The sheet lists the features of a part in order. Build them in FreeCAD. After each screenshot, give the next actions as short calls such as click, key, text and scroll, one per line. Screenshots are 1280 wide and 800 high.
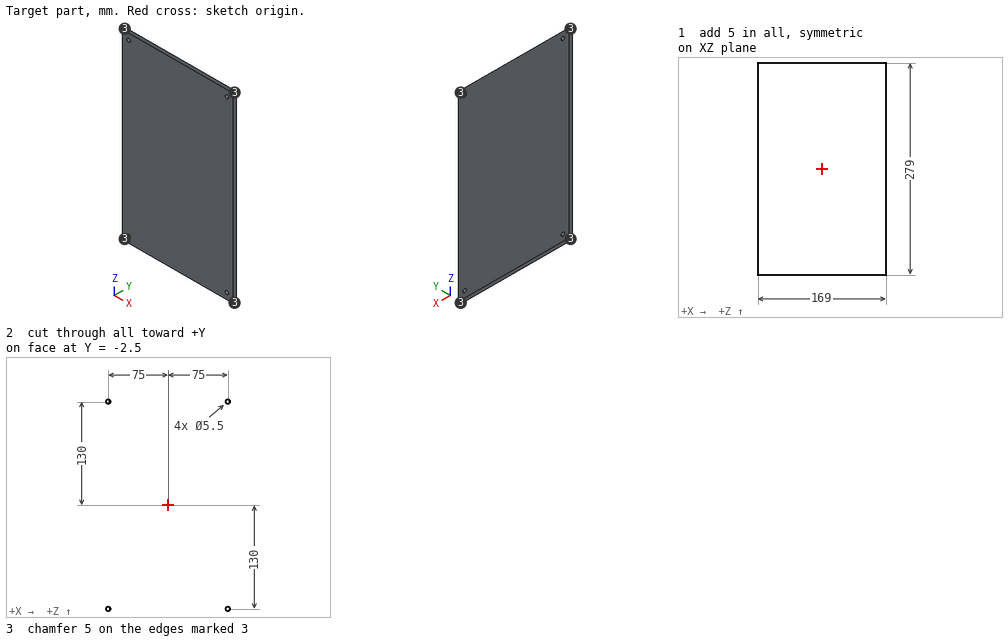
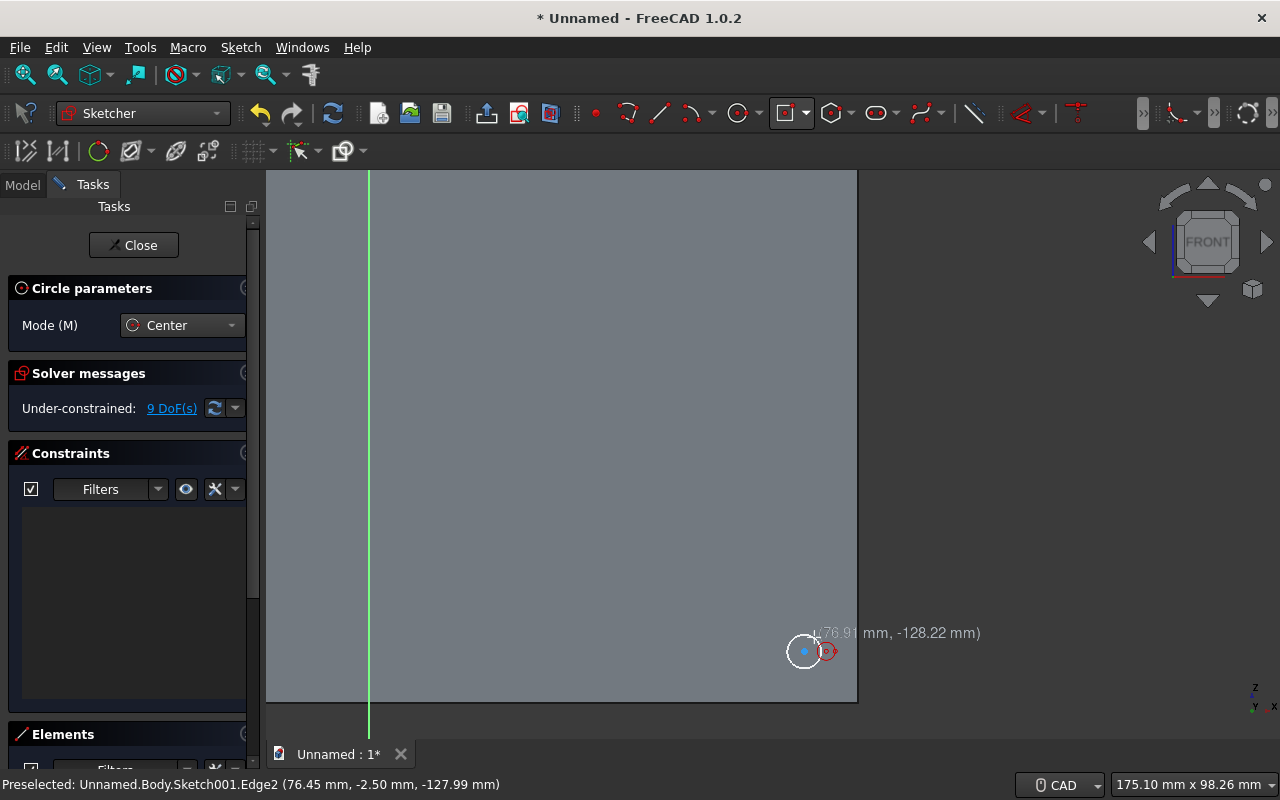
scroll(814, 637, down, 7)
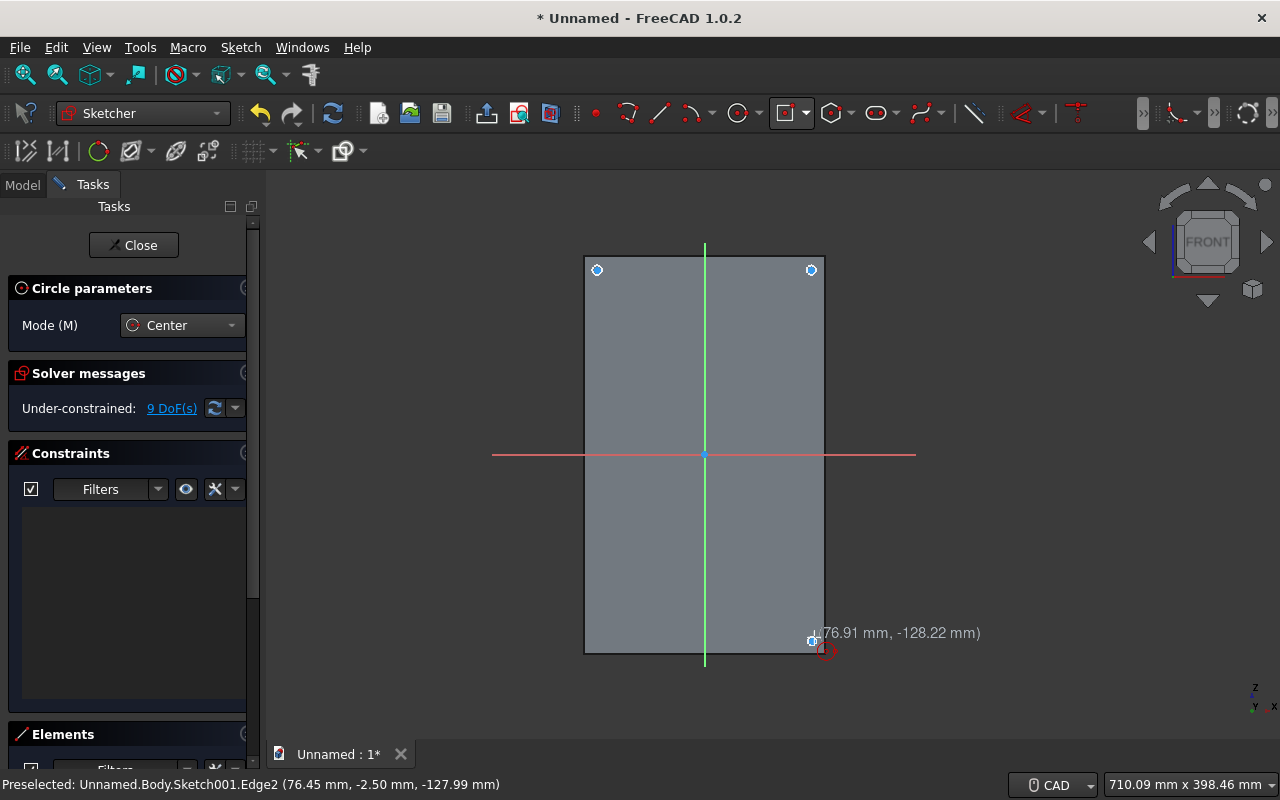
scroll(597, 640, up, 9)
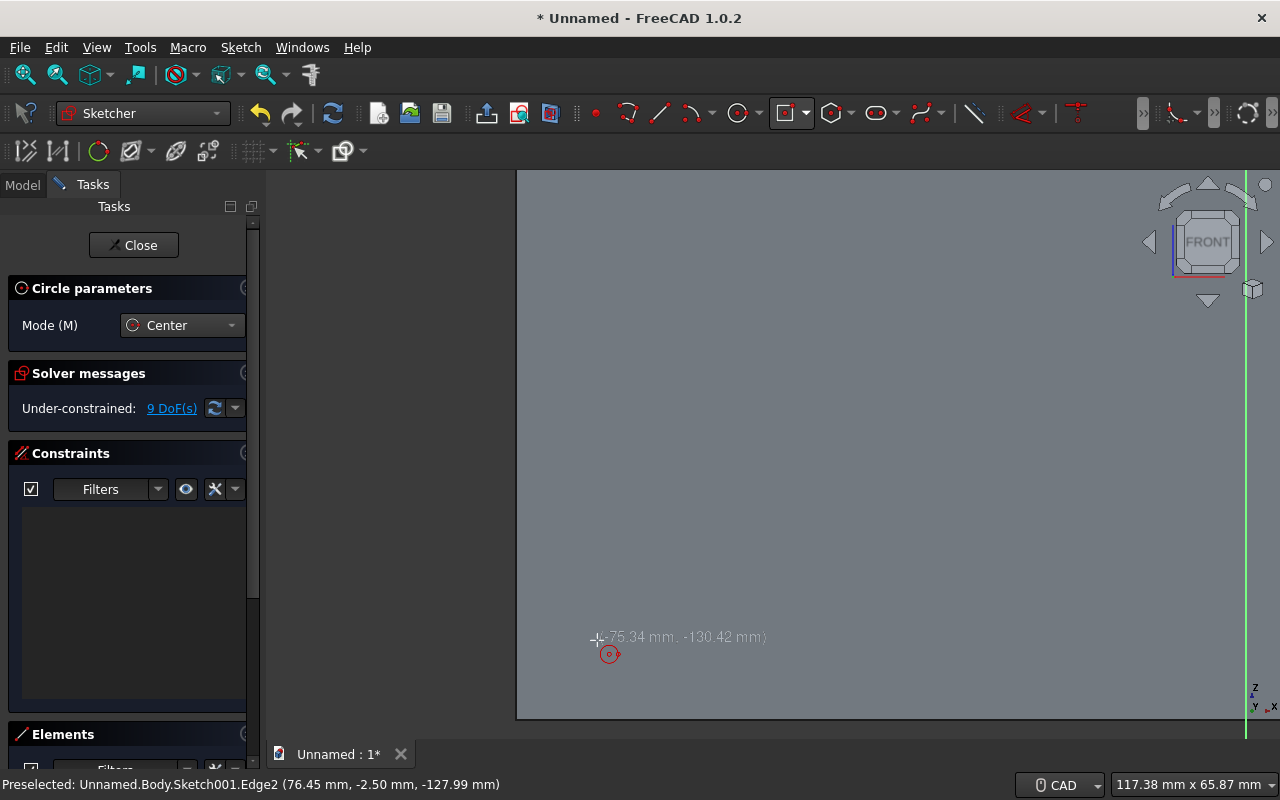
scroll(597, 641, down, 9)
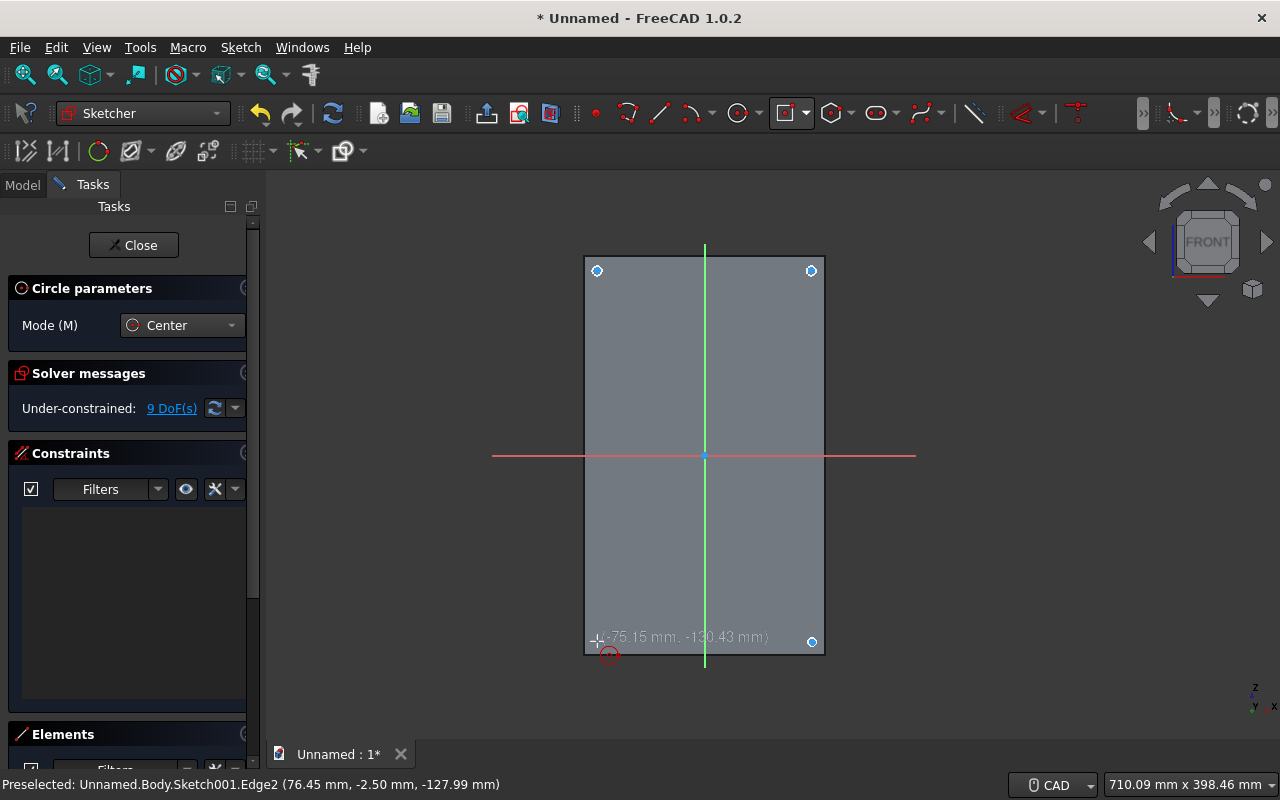
click(597, 641)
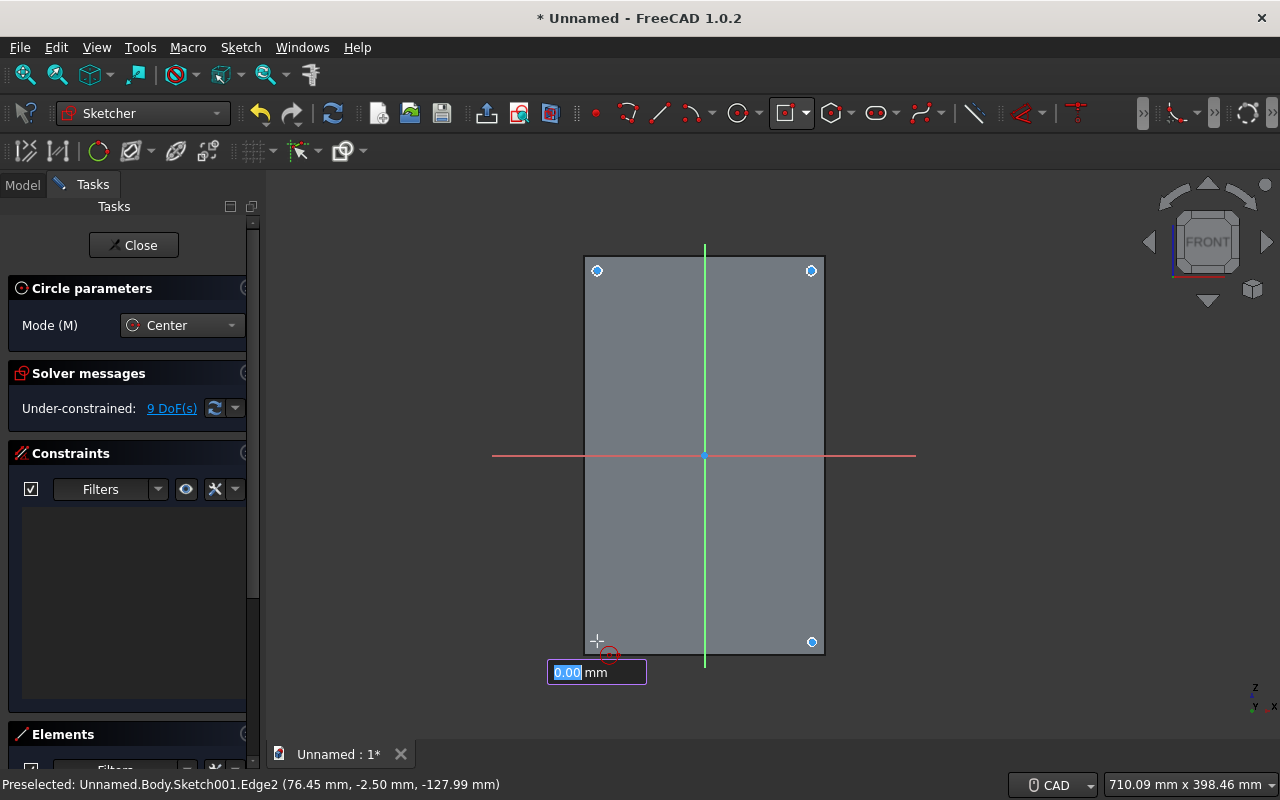
scroll(600, 638, up, 7)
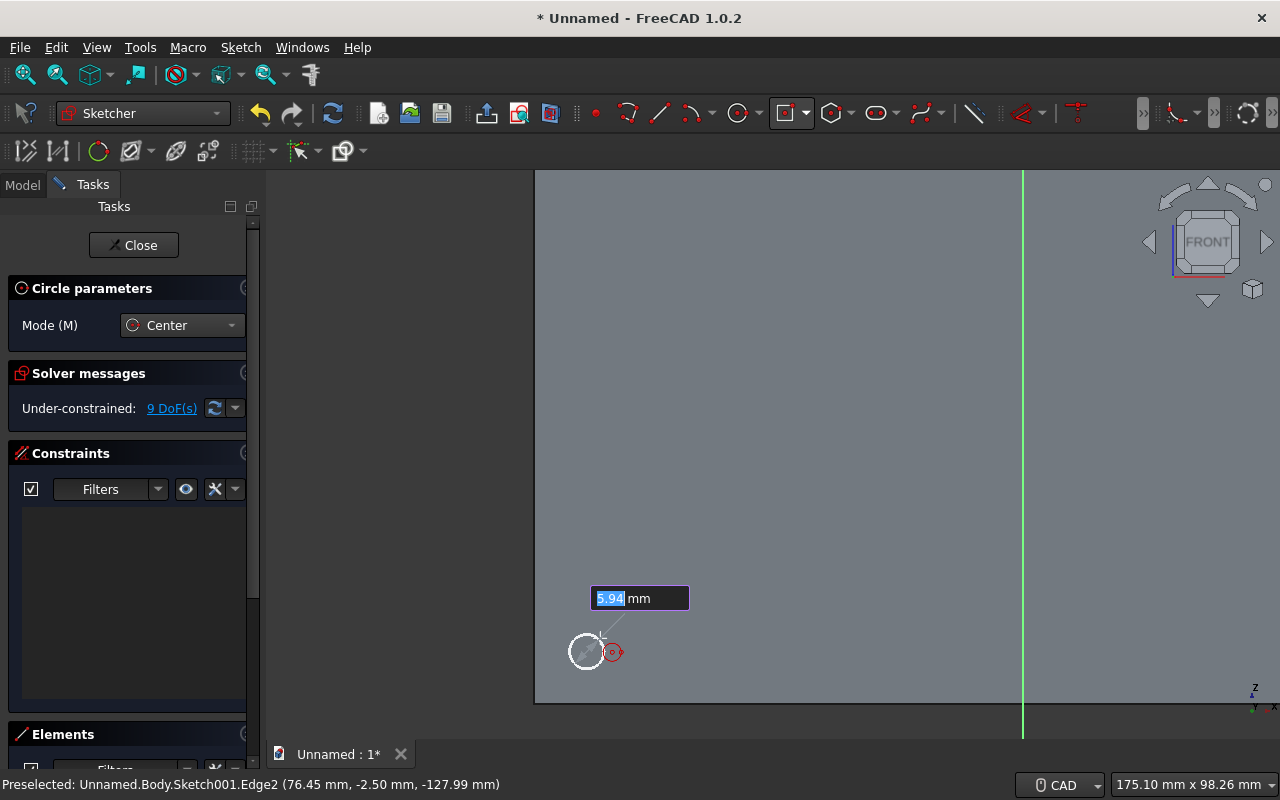
click(600, 637)
key(Escape)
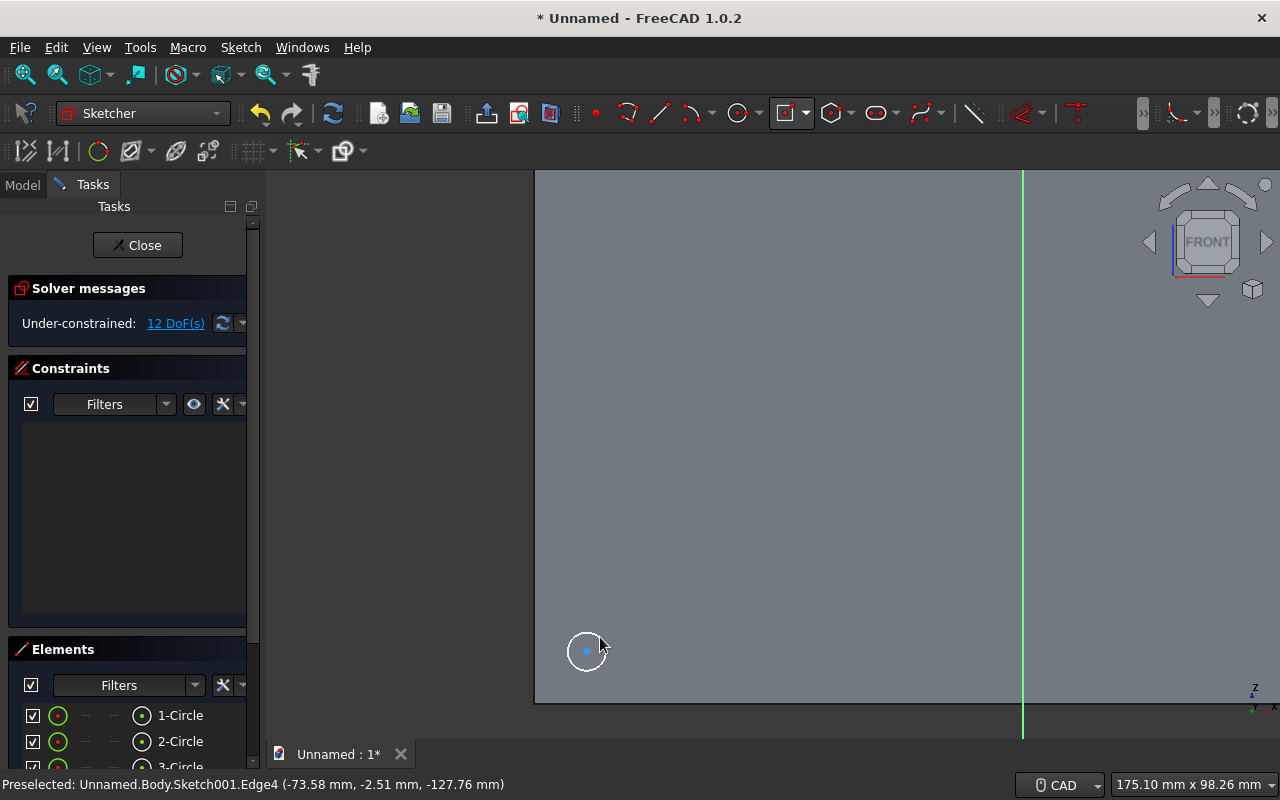
scroll(600, 637, down, 7)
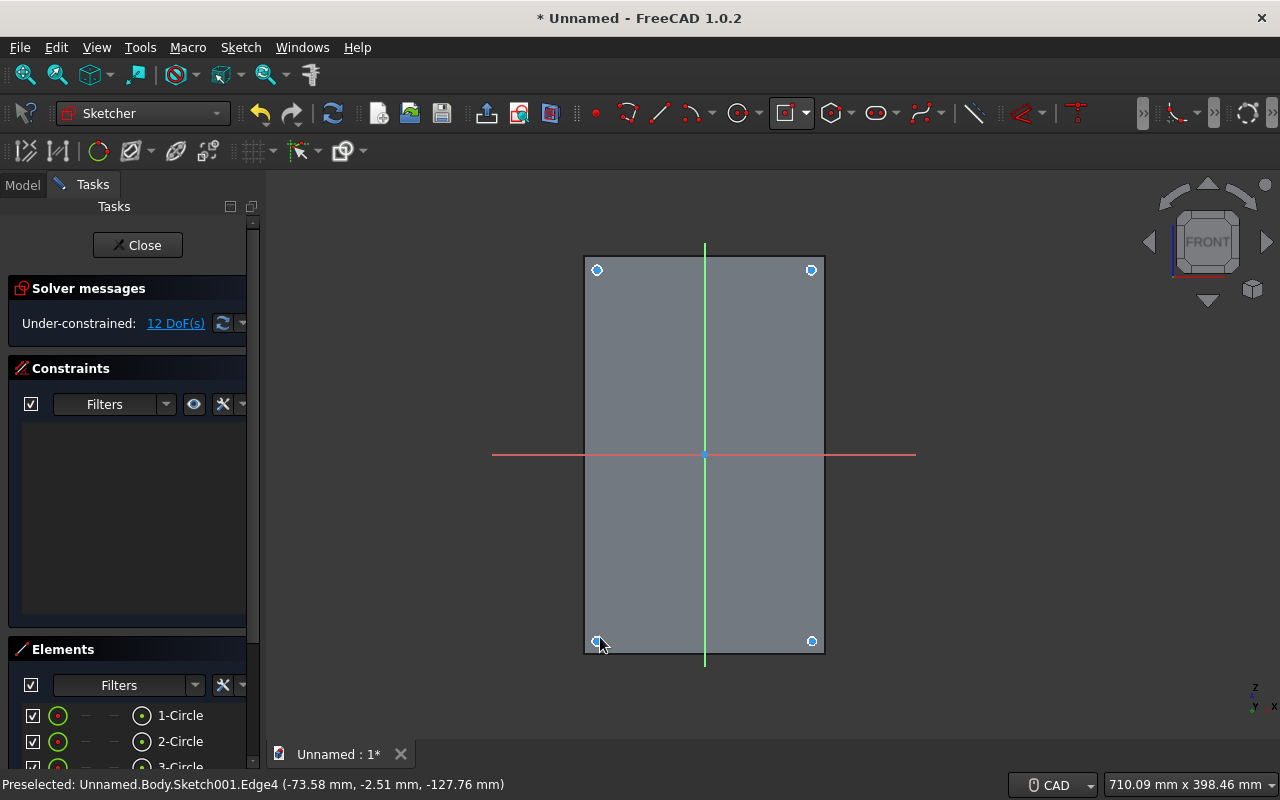
scroll(600, 267, up, 6)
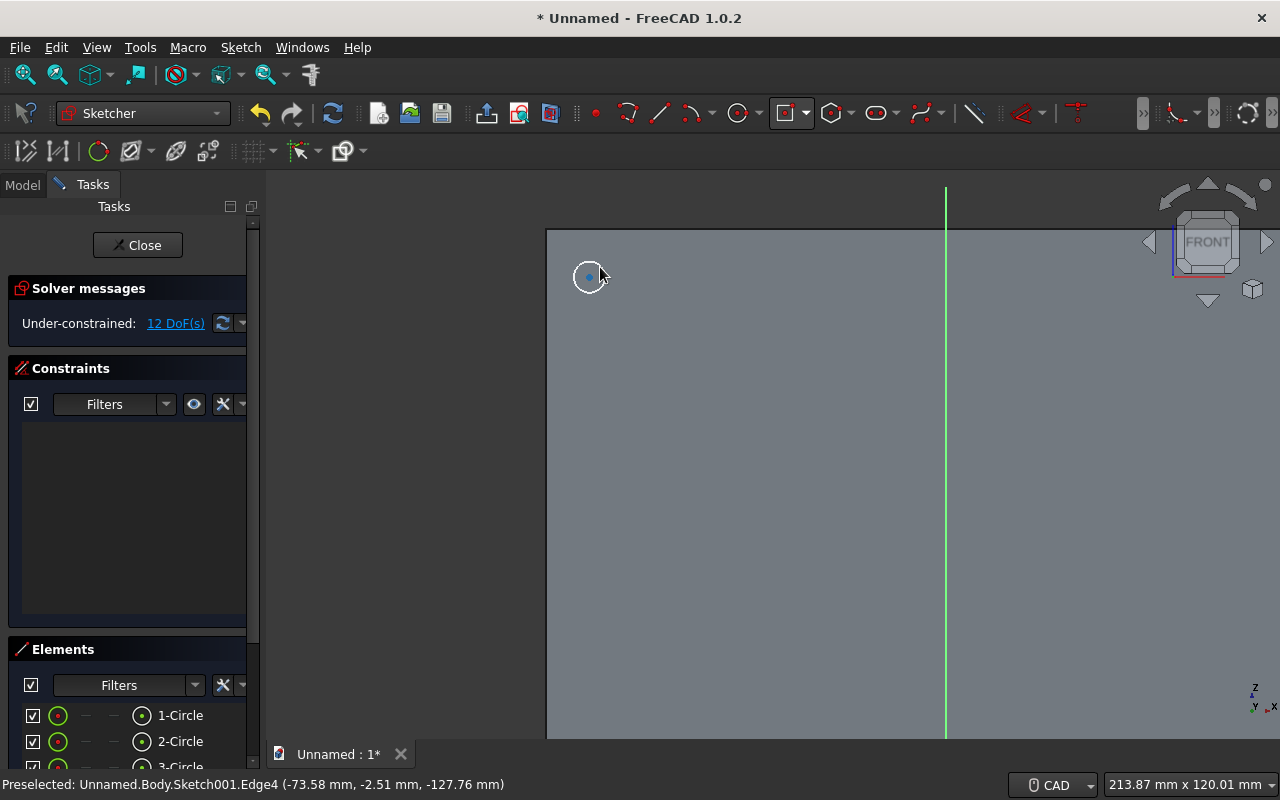
click(601, 266)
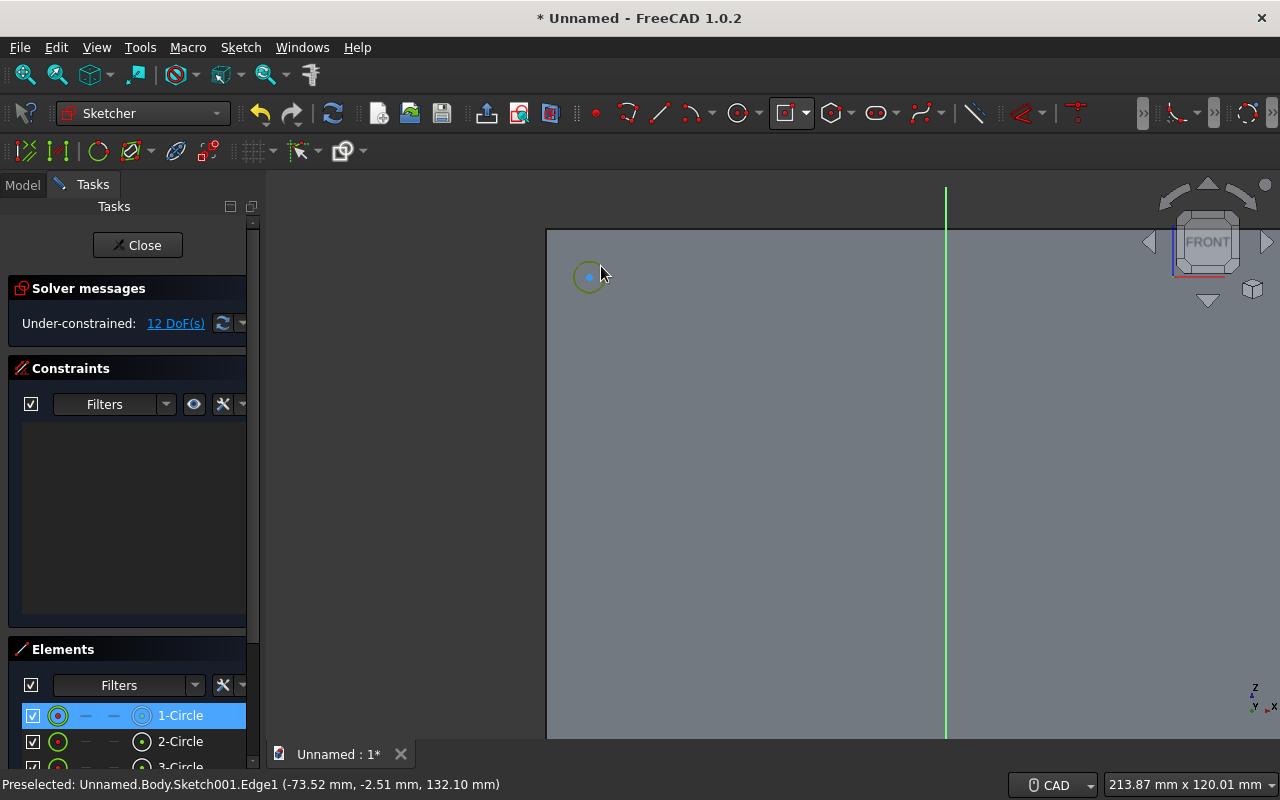
scroll(600, 267, down, 6)